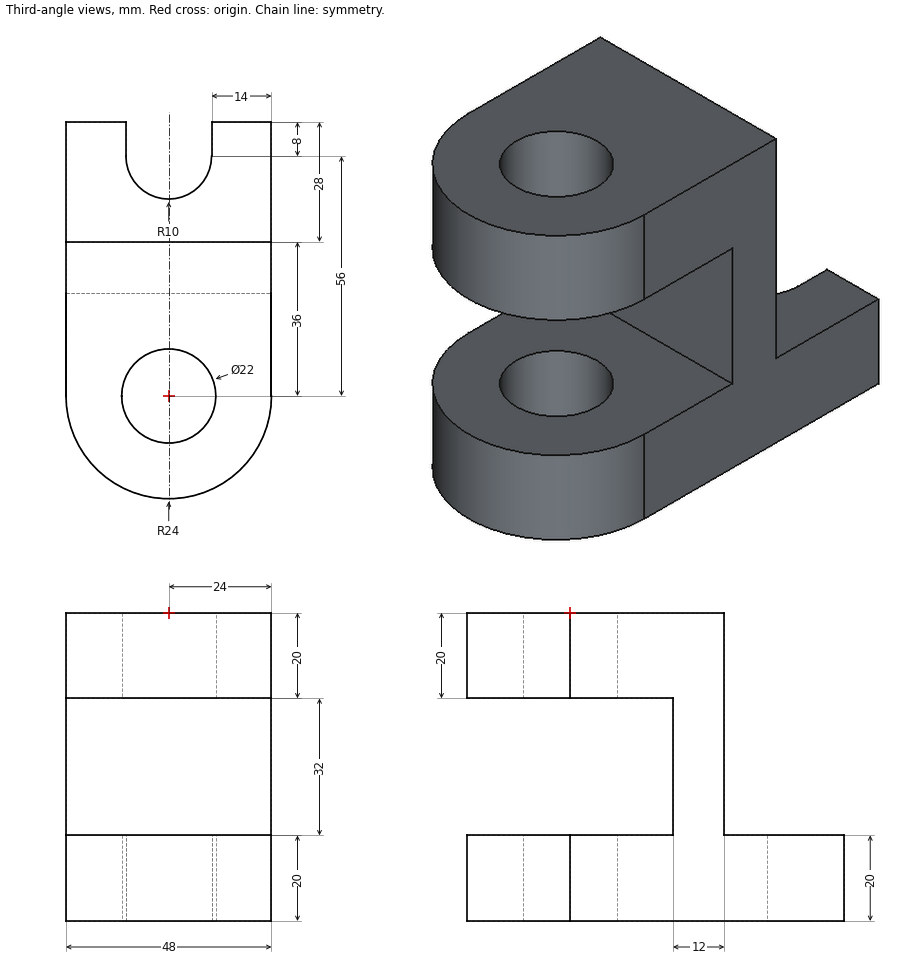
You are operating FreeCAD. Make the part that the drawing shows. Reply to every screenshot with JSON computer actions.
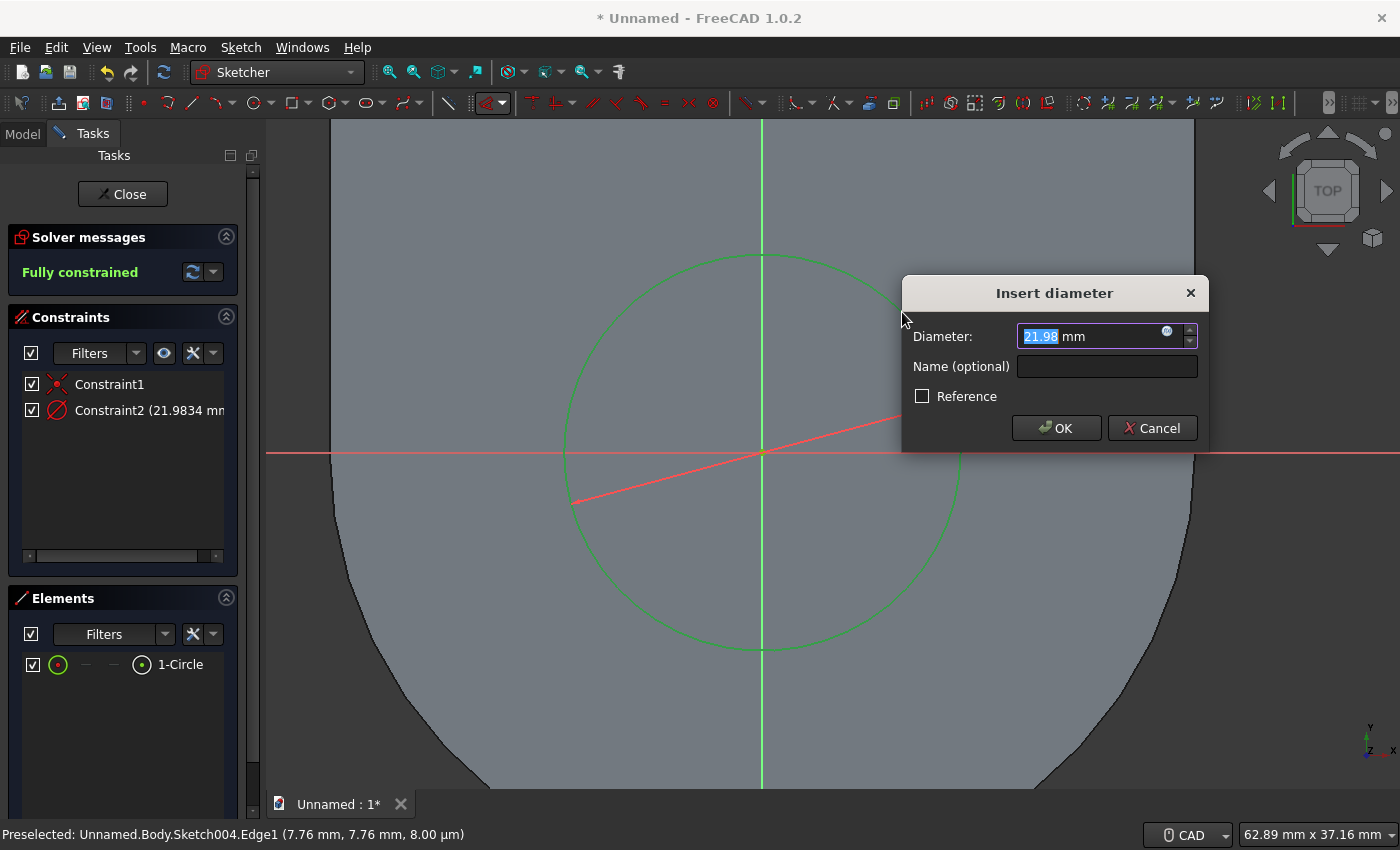
{"action": "type", "text": "22"}
{"action": "key", "text": "Return"}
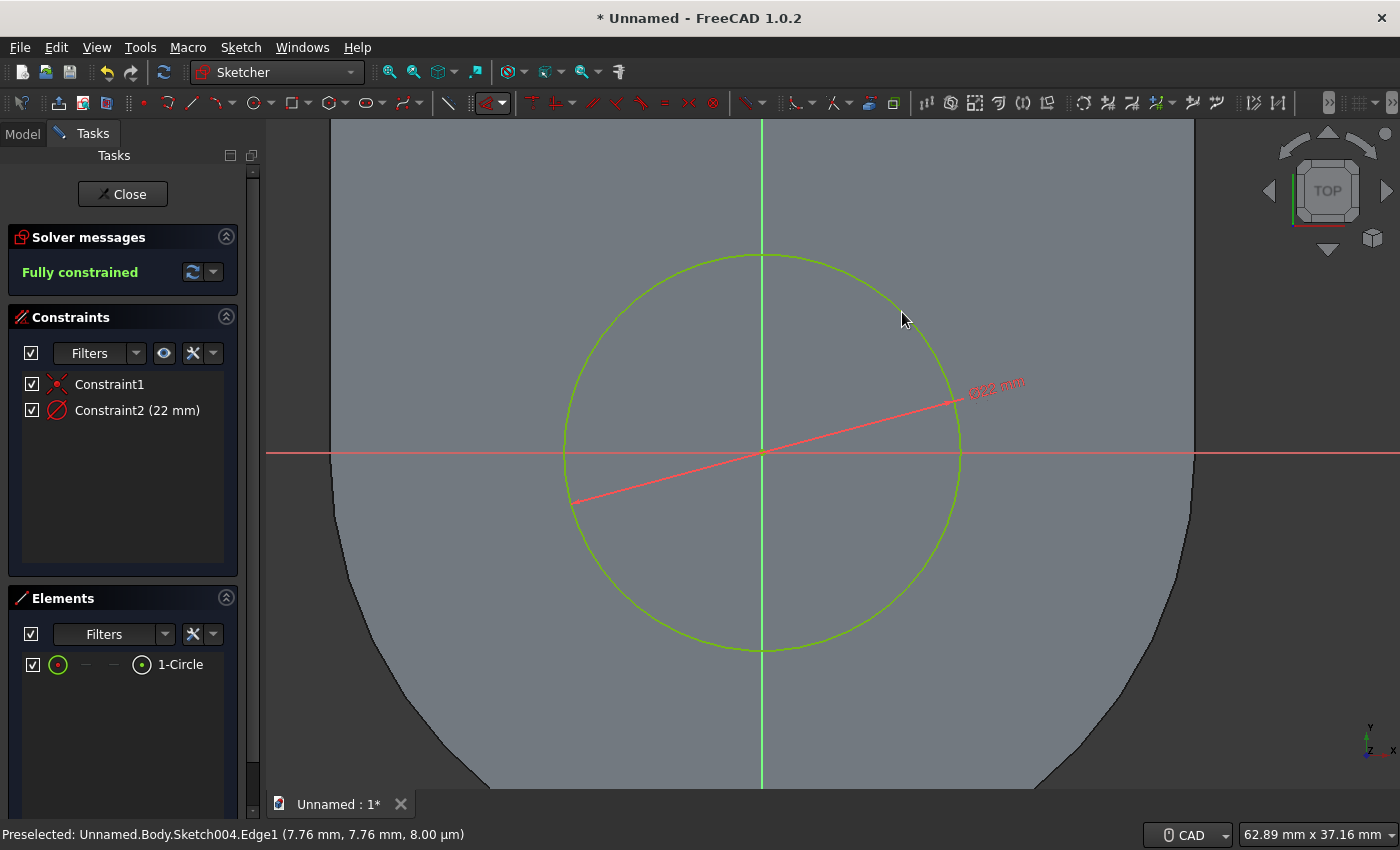
{"action": "left_click", "coordinate": [123, 194]}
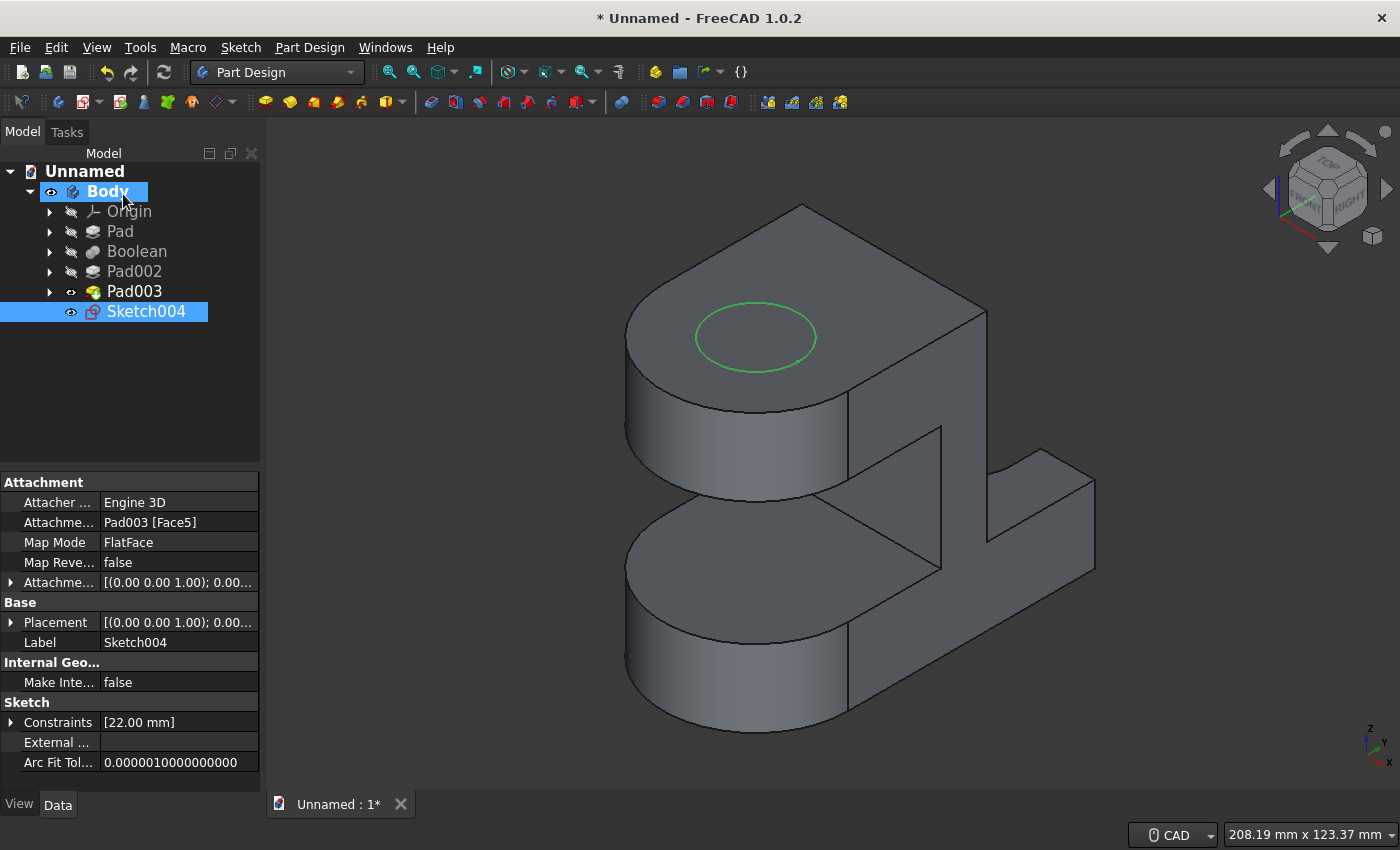
{"action": "left_click", "coordinate": [432, 102]}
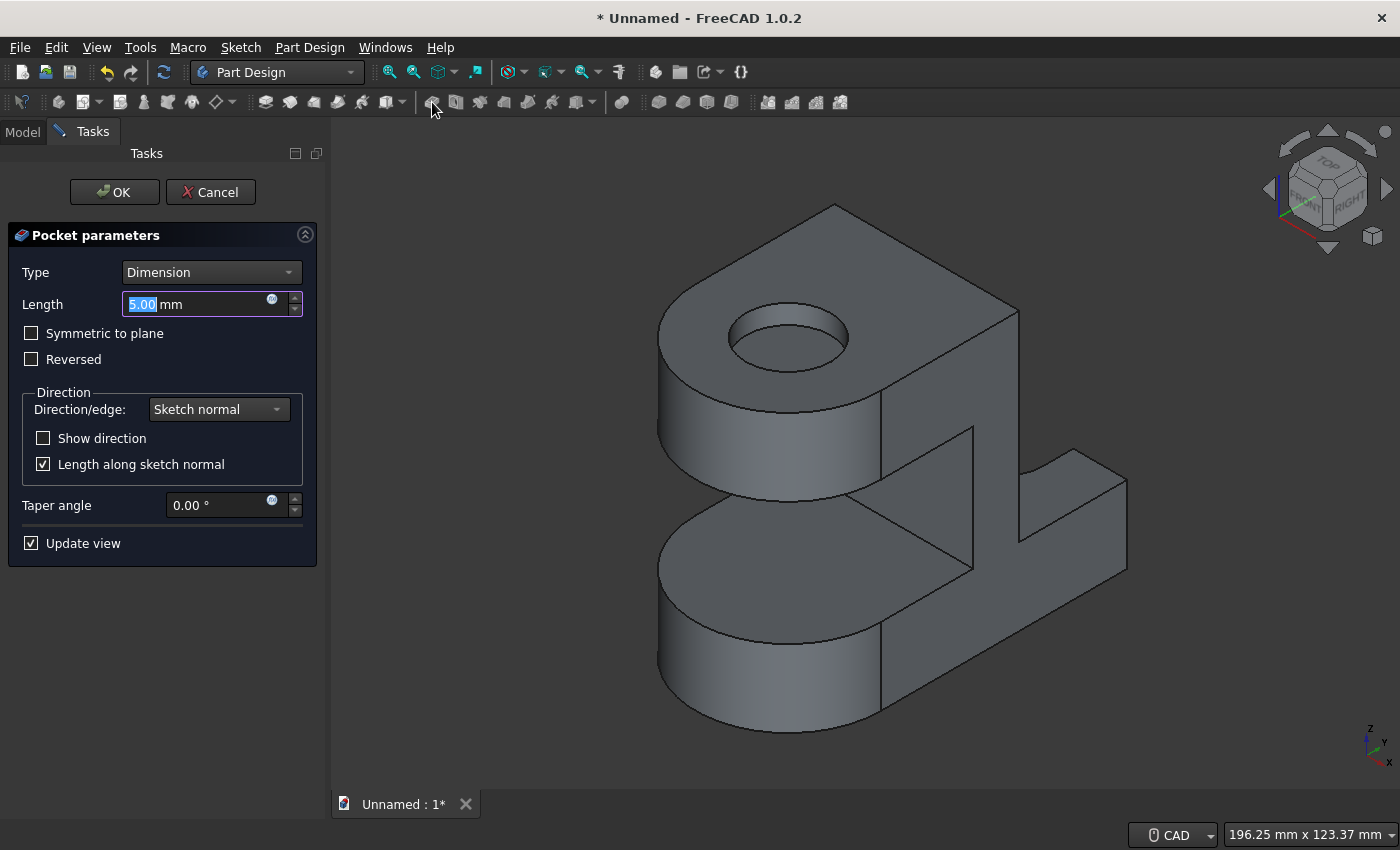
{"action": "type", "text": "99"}
{"action": "key", "text": "Tab"}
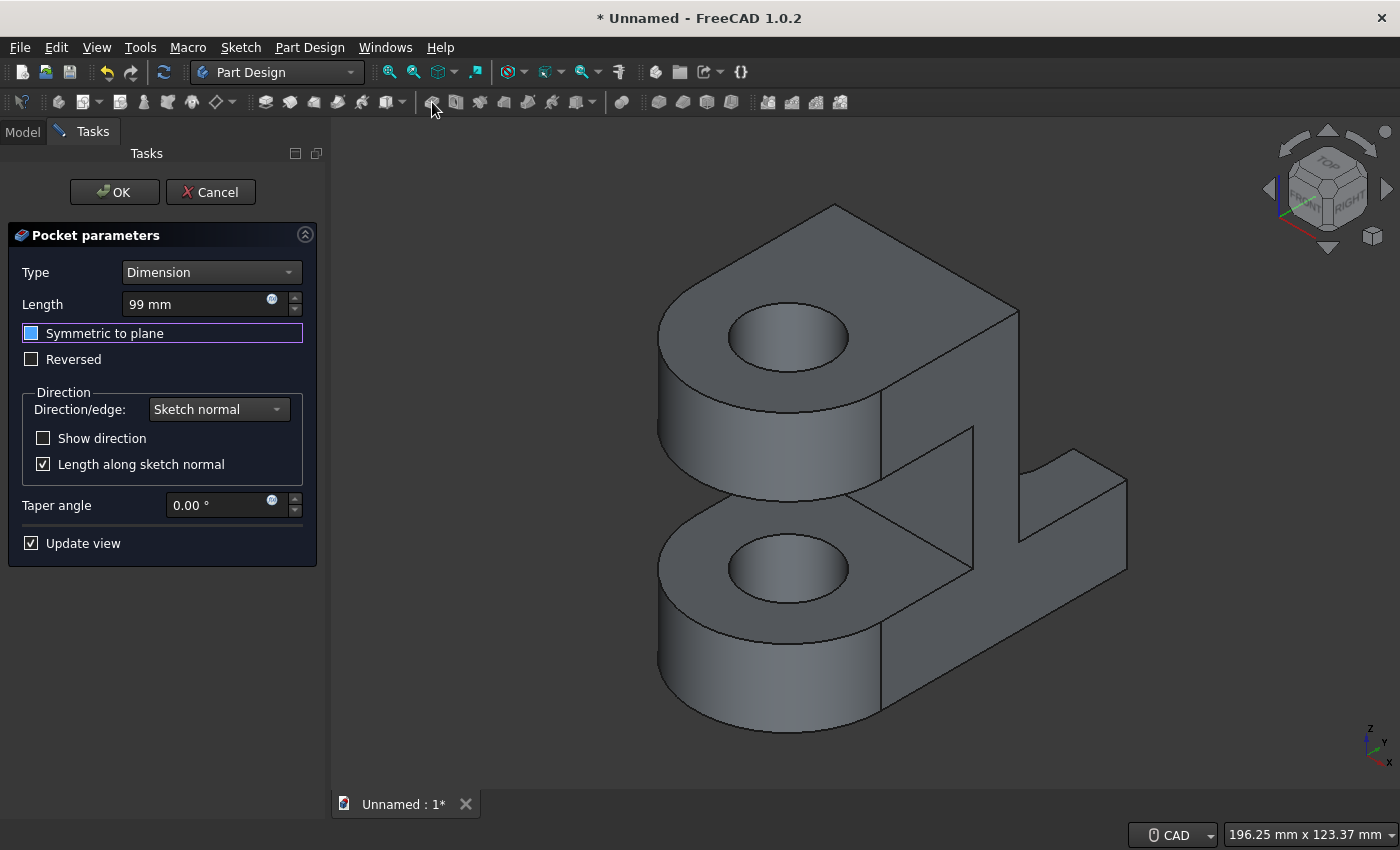
{"action": "left_click", "coordinate": [115, 192]}